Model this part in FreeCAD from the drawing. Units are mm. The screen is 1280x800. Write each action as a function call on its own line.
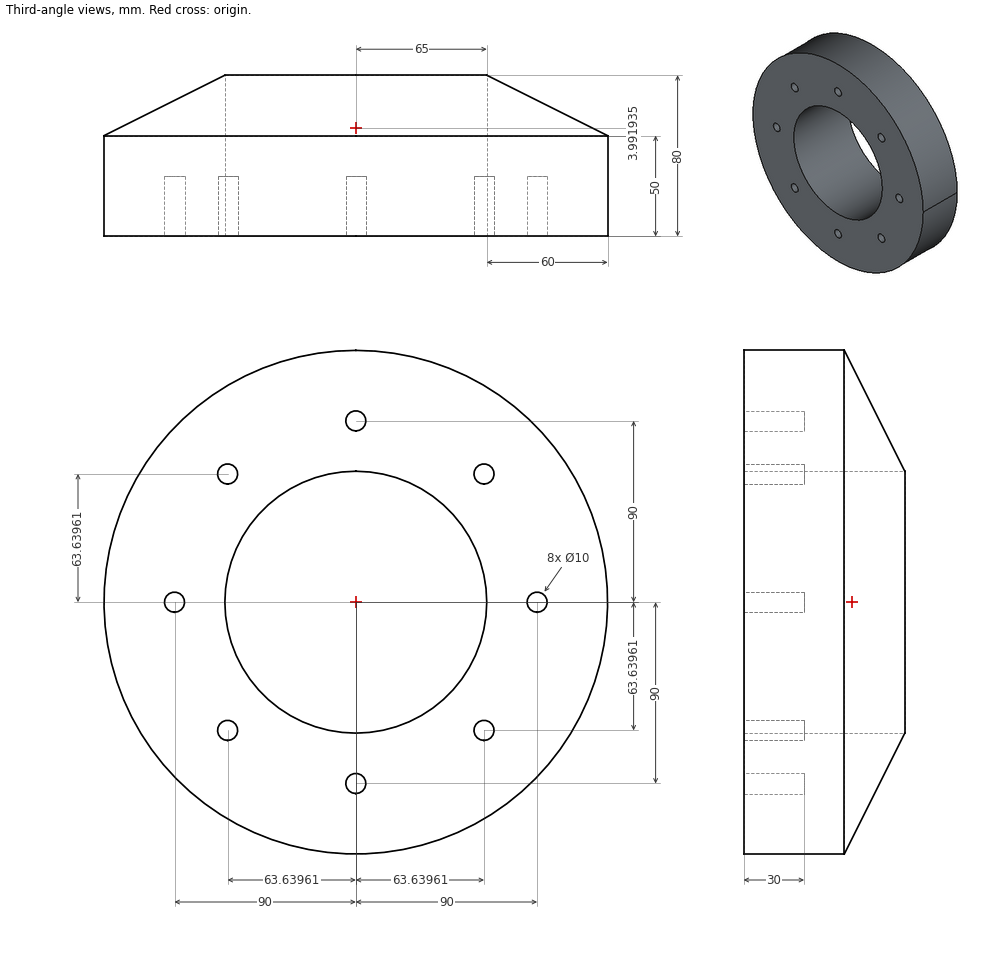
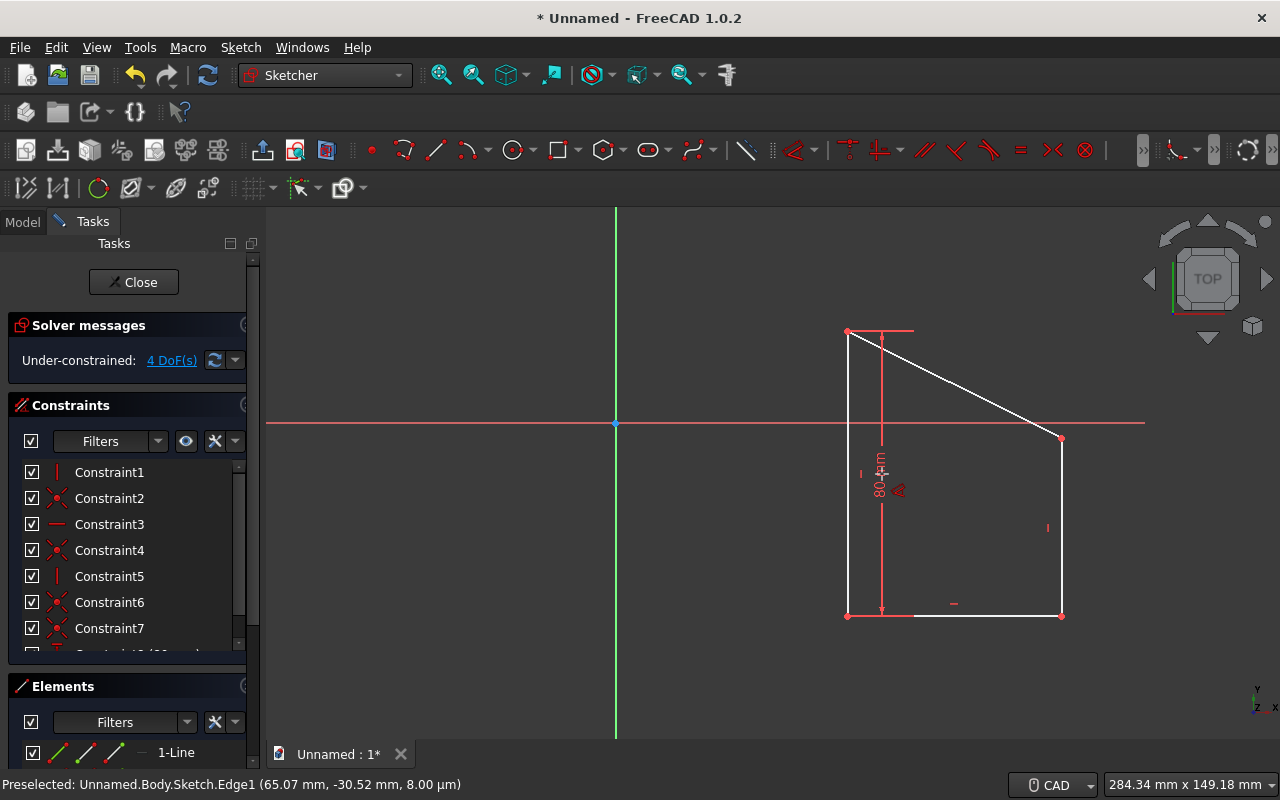
click(912, 616)
click(955, 650)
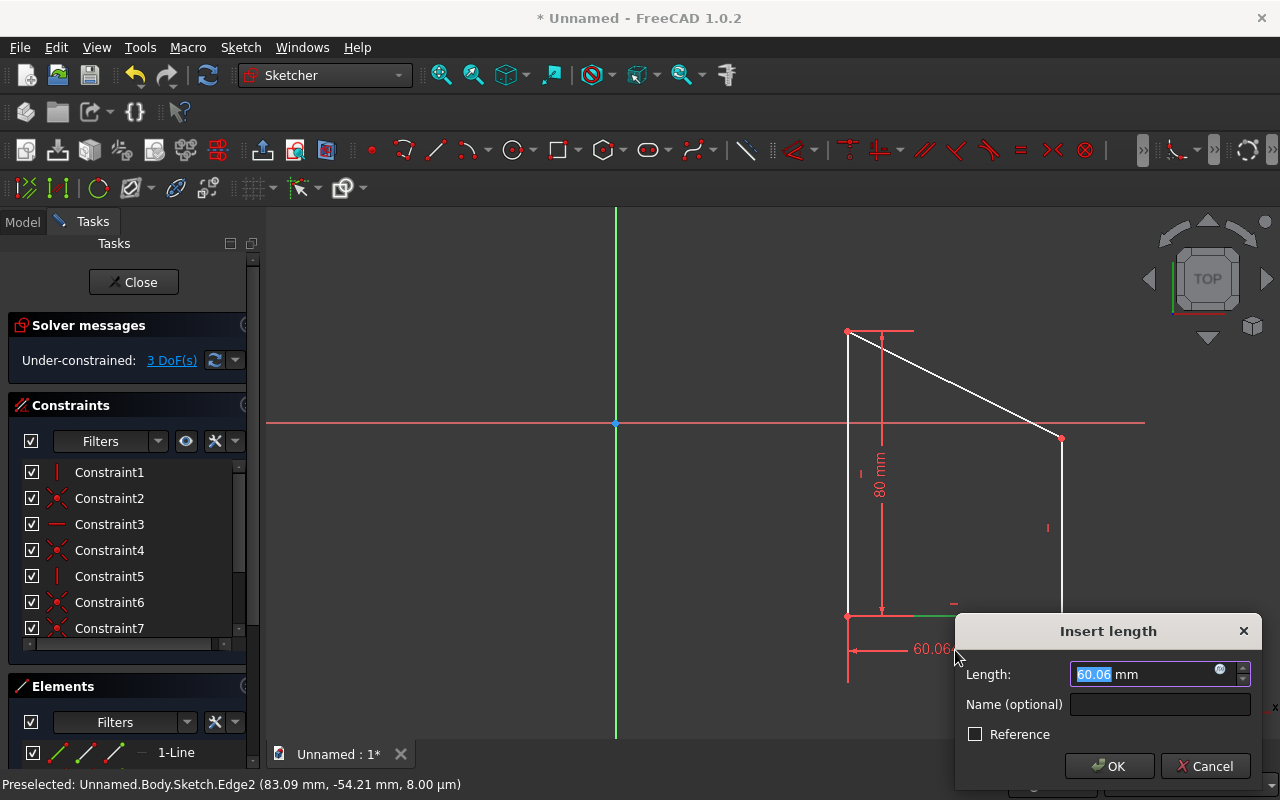
text(60)
key(Return)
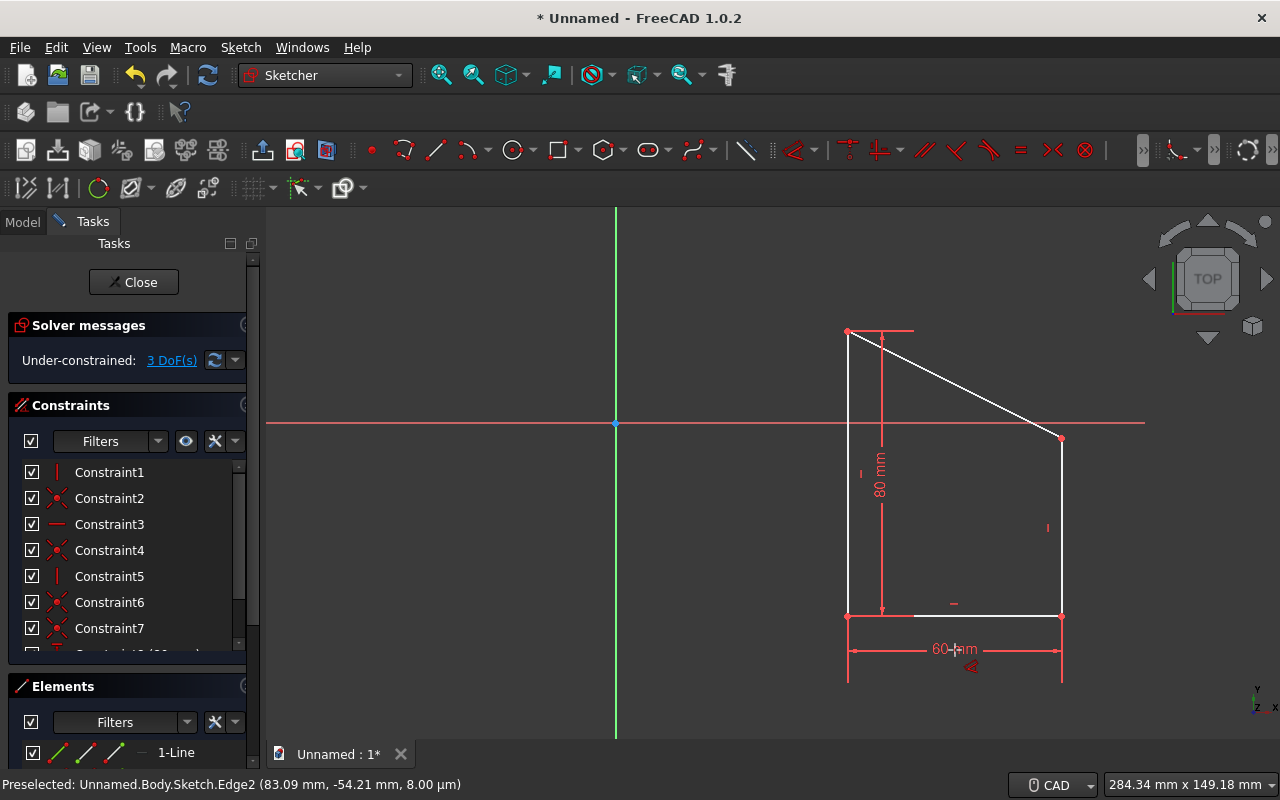
click(1062, 563)
click(1096, 527)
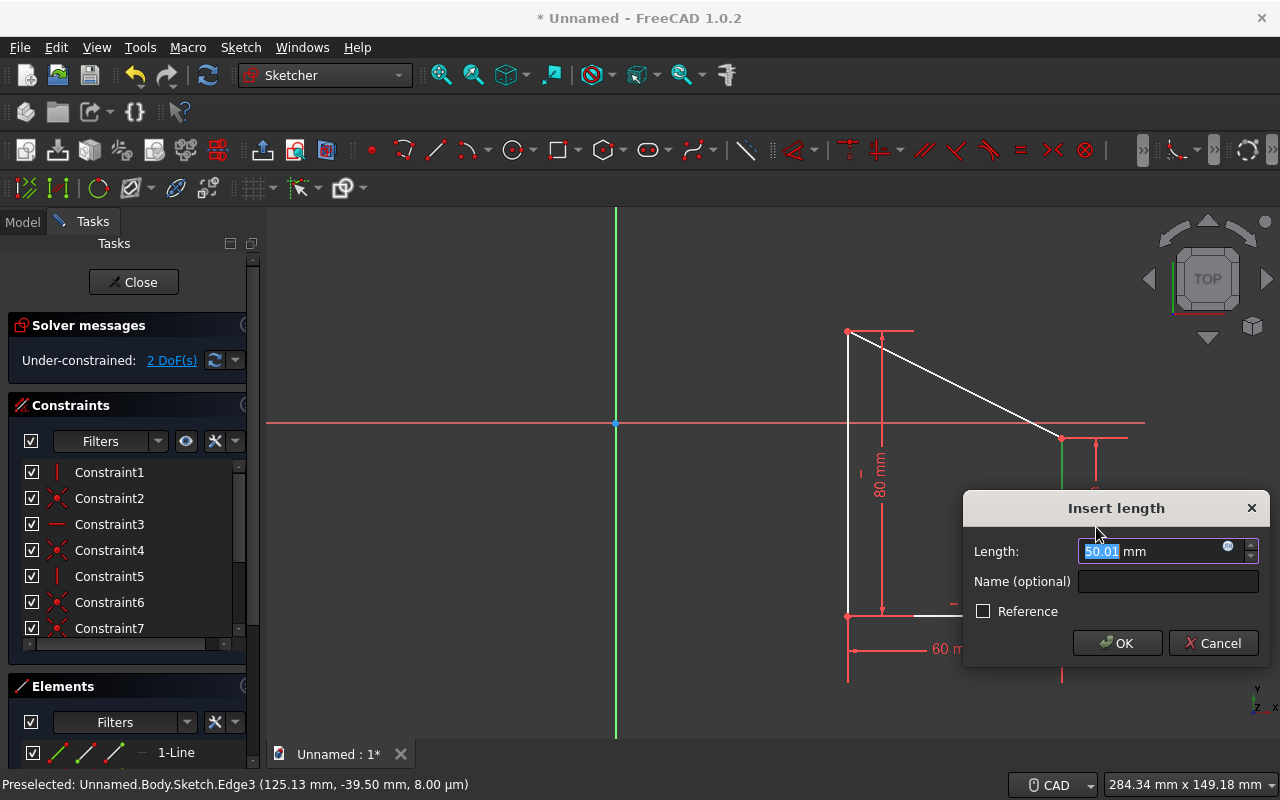
text(50)
key(Return)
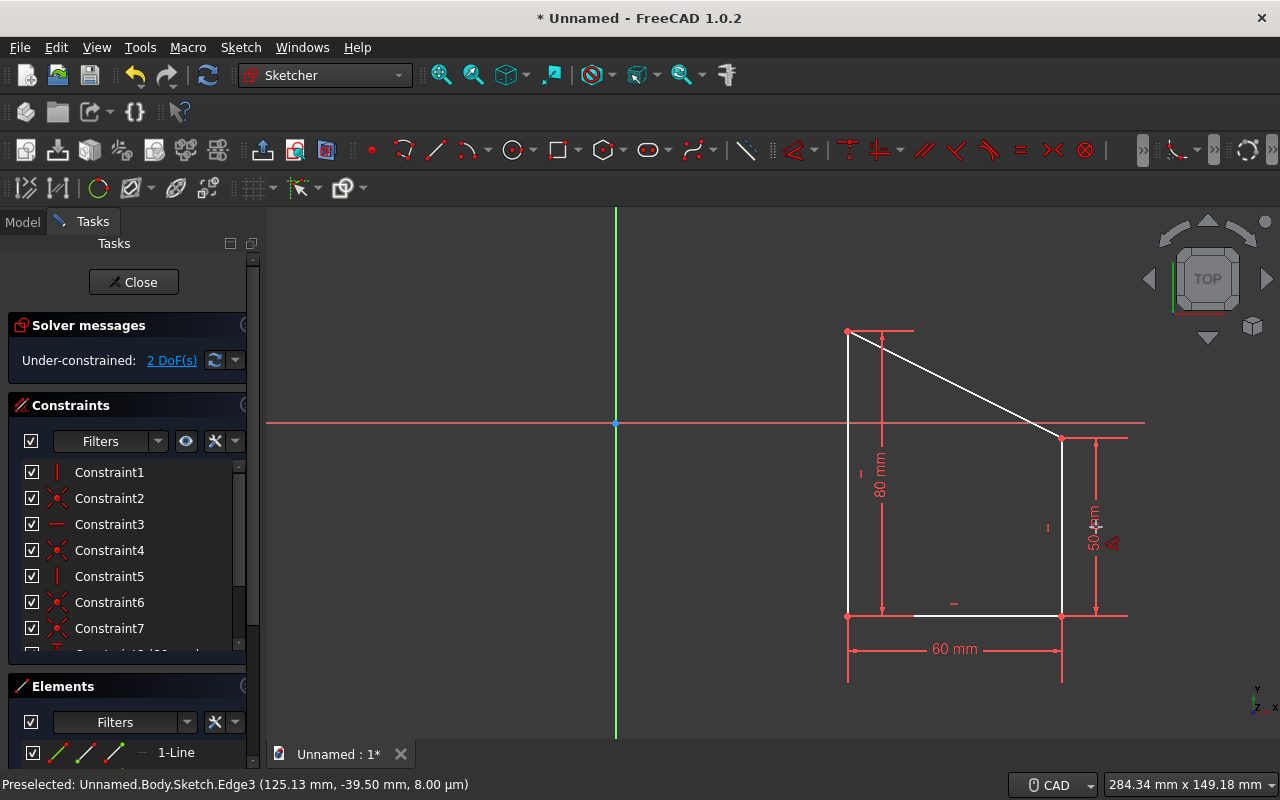
click(848, 331)
click(732, 297)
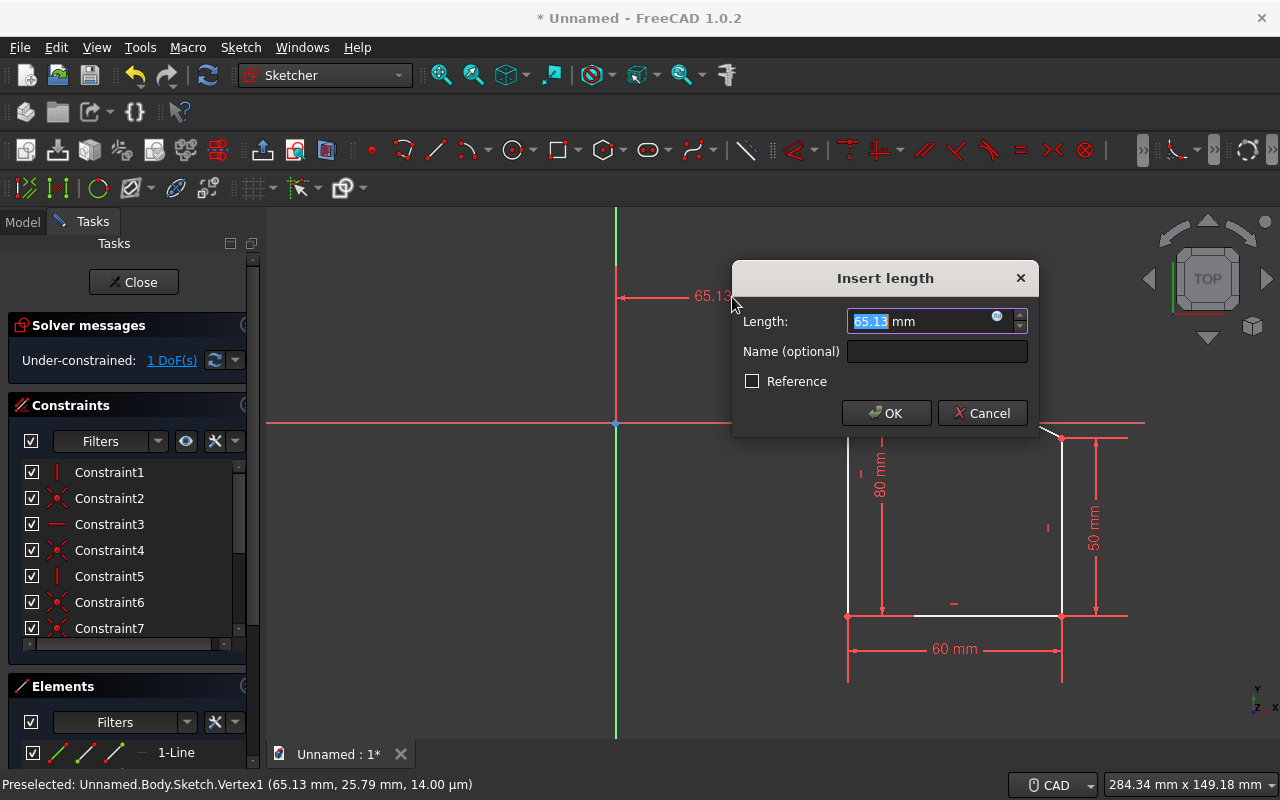
text(65)
key(Return)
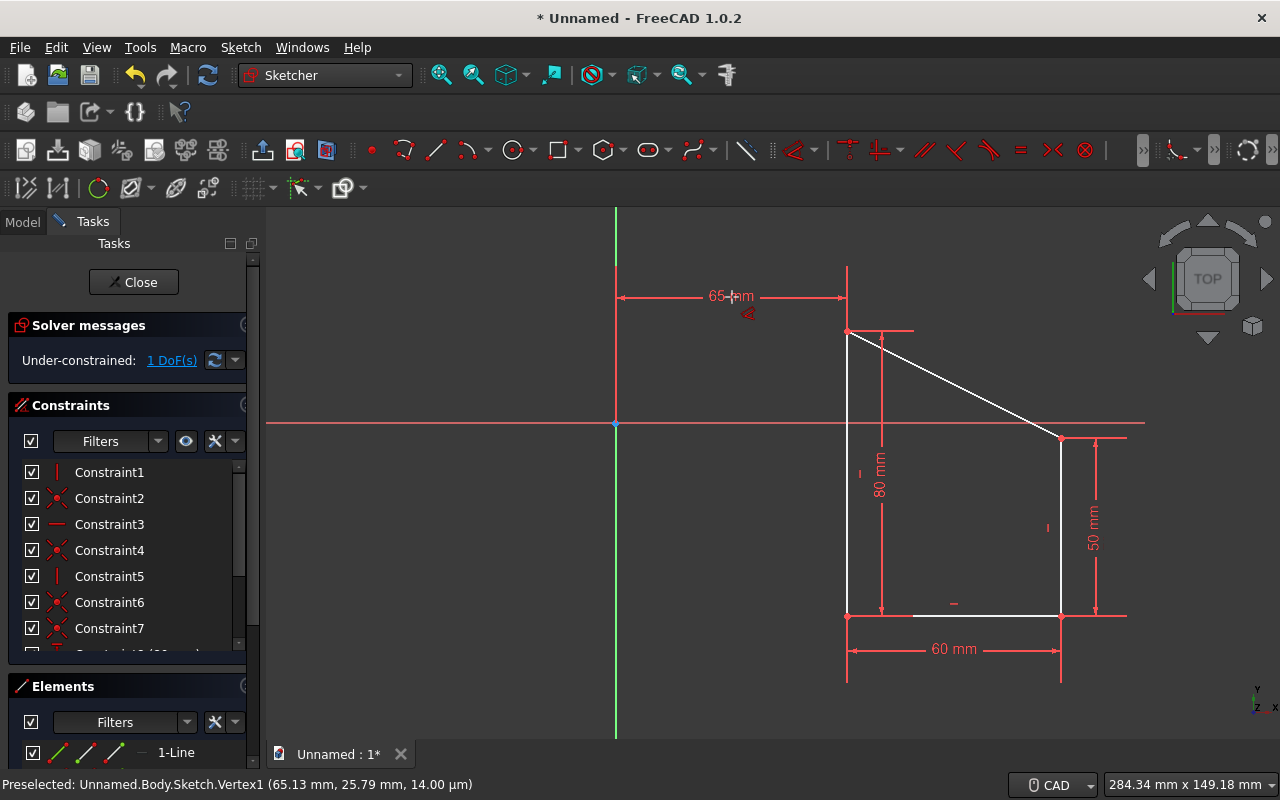
scroll(1061, 438, up, 6)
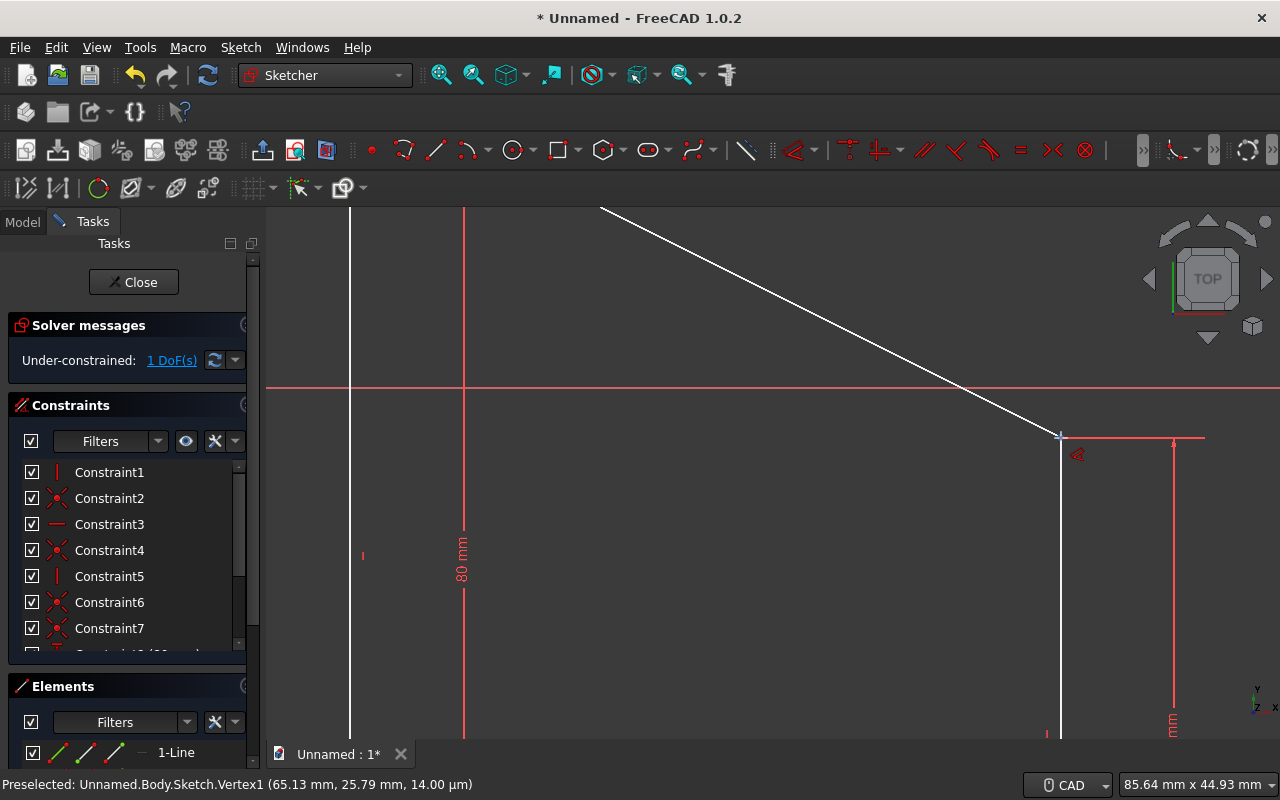
click(1061, 438)
click(1095, 413)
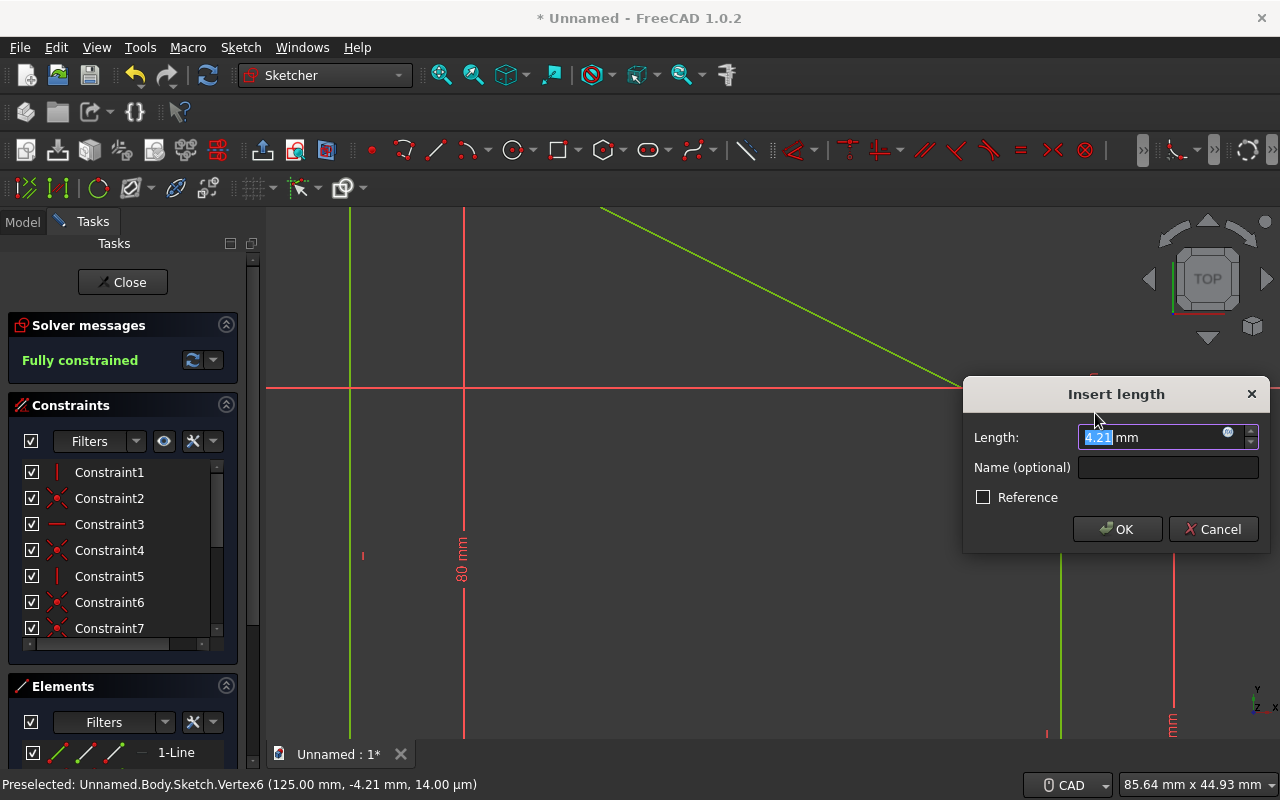
text(3.991935)
key(Return)
key(Escape)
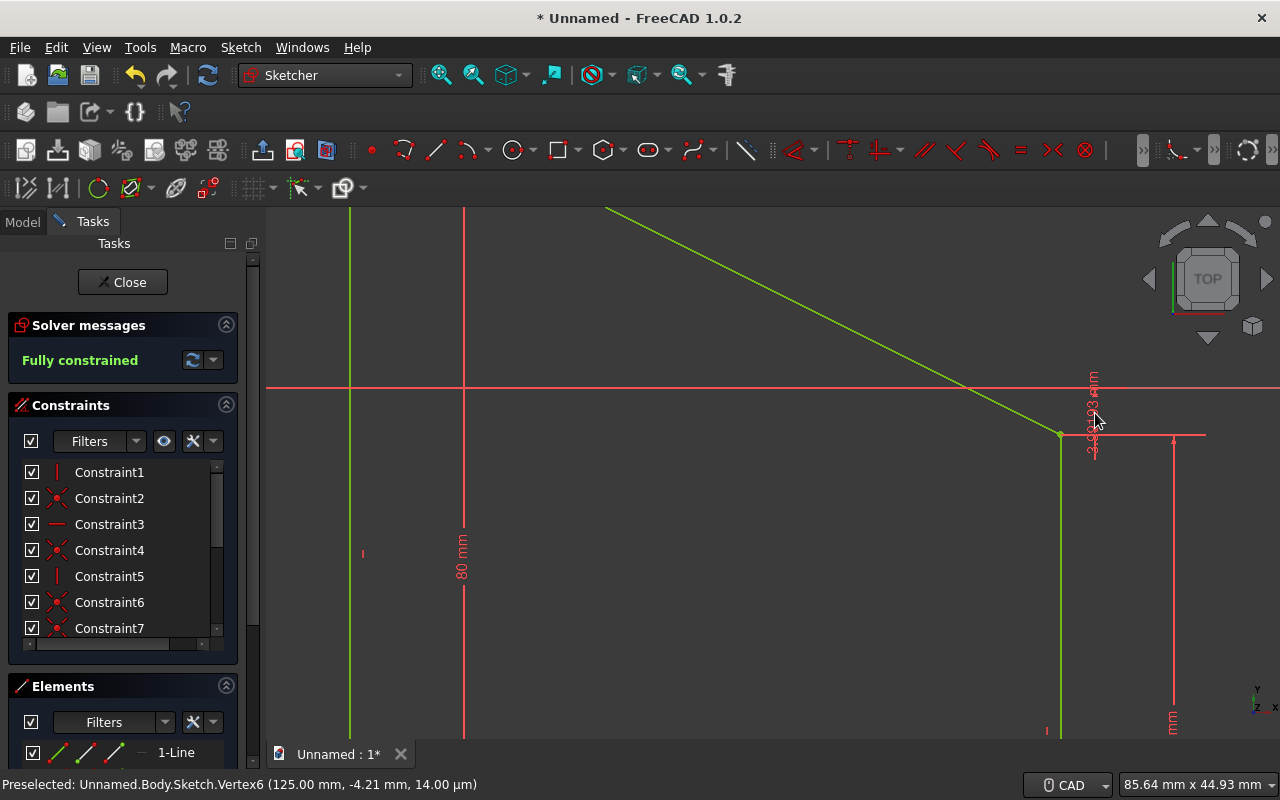
click(123, 282)